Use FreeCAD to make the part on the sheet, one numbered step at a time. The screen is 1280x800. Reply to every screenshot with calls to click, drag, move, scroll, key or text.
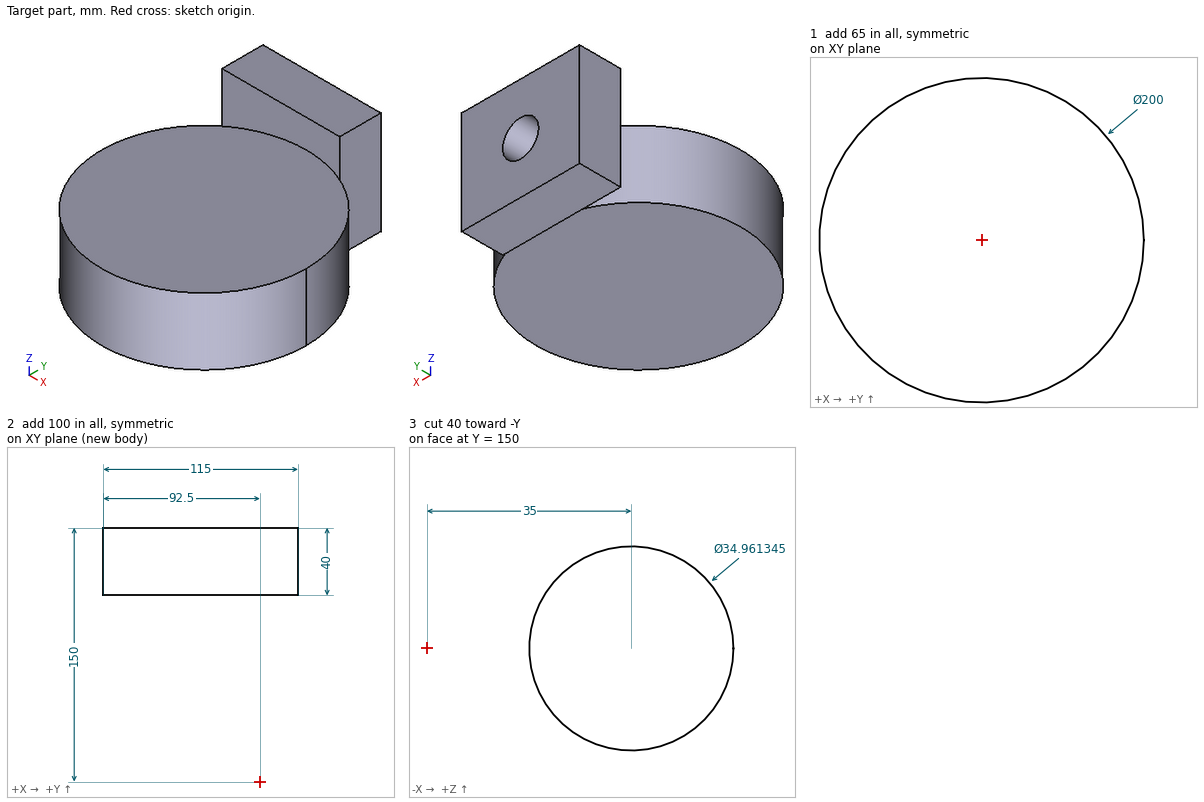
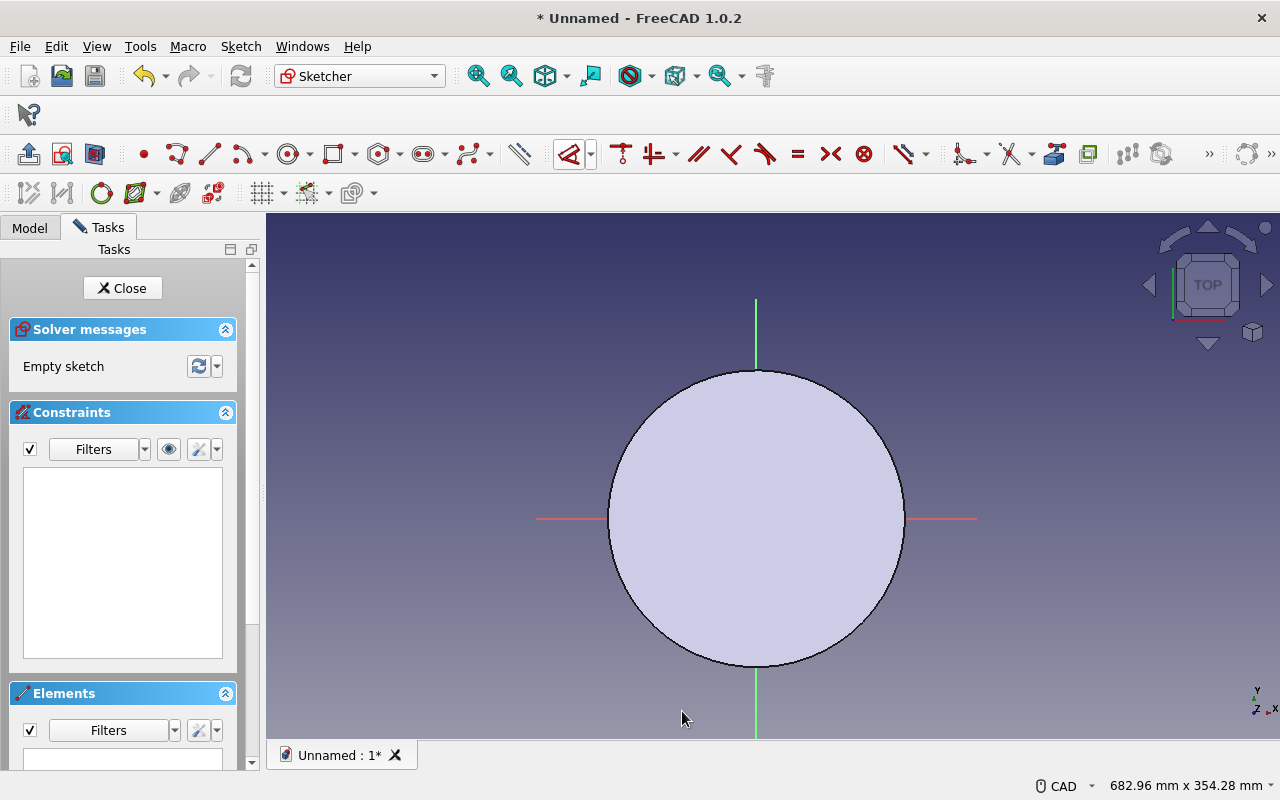
scroll(705, 268, up, 2)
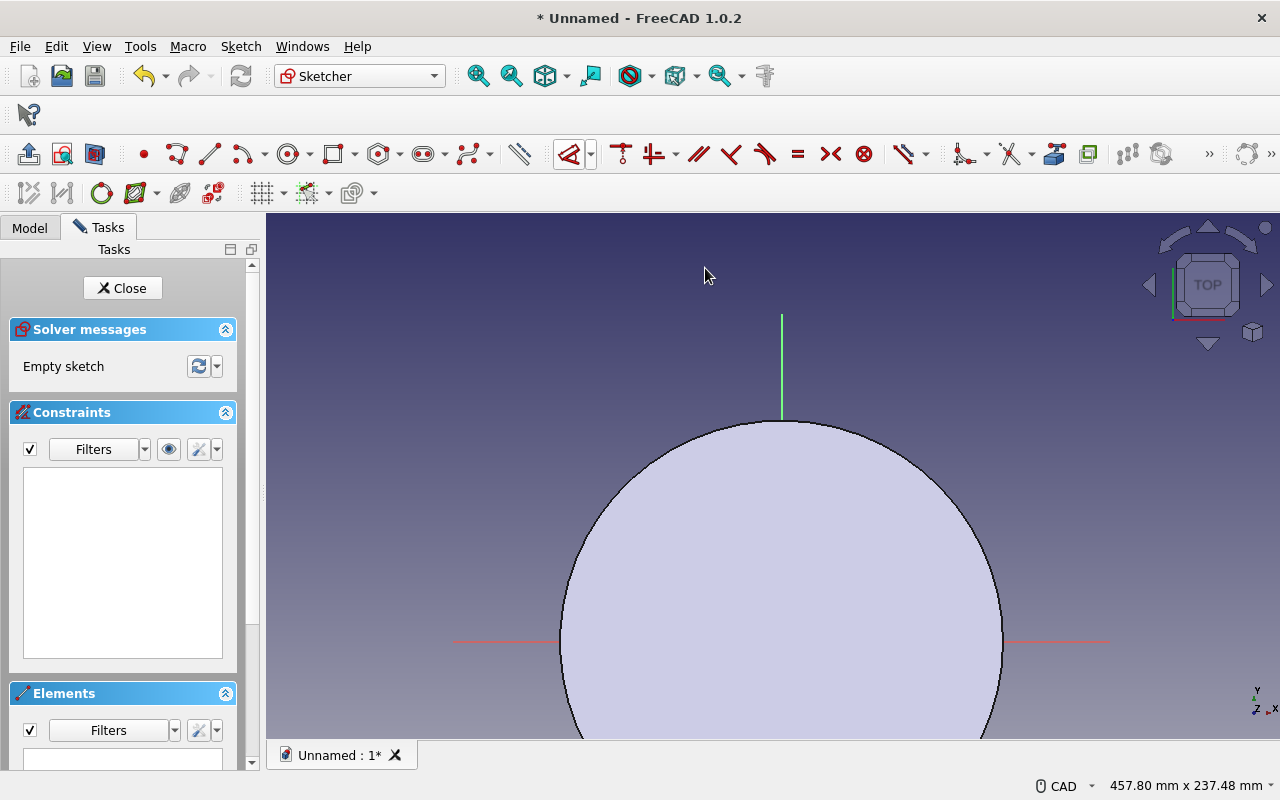
key(g)
key(r)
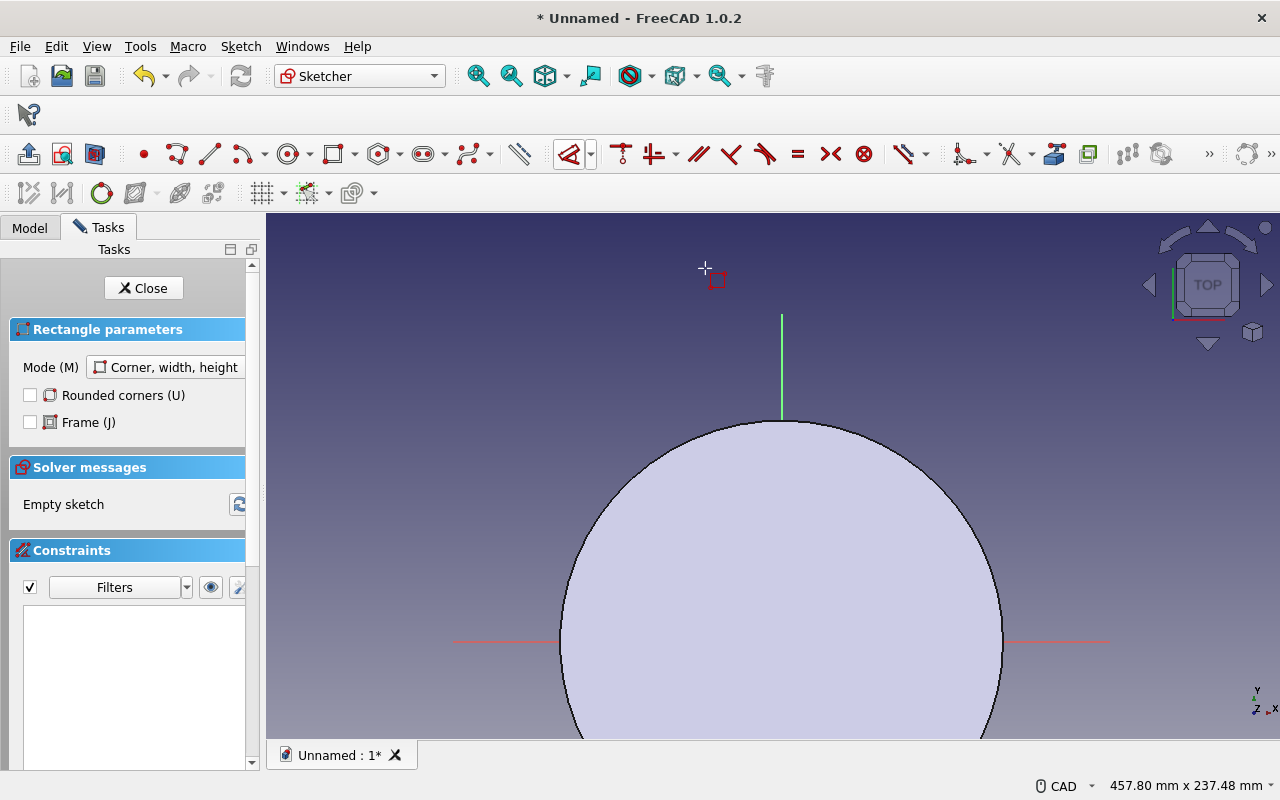
click(577, 310)
move(831, 398)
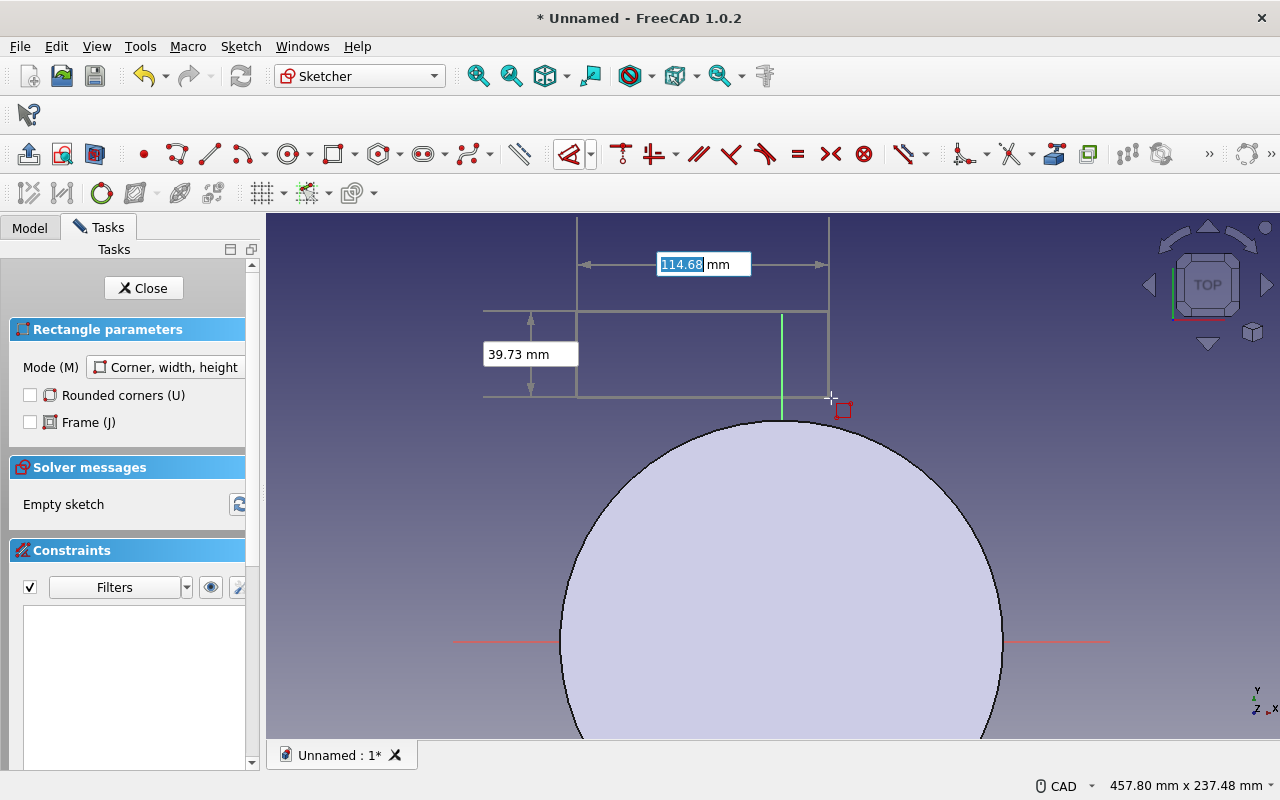
text(115)
key(Tab)
text(40)
key(Return)
key(Escape)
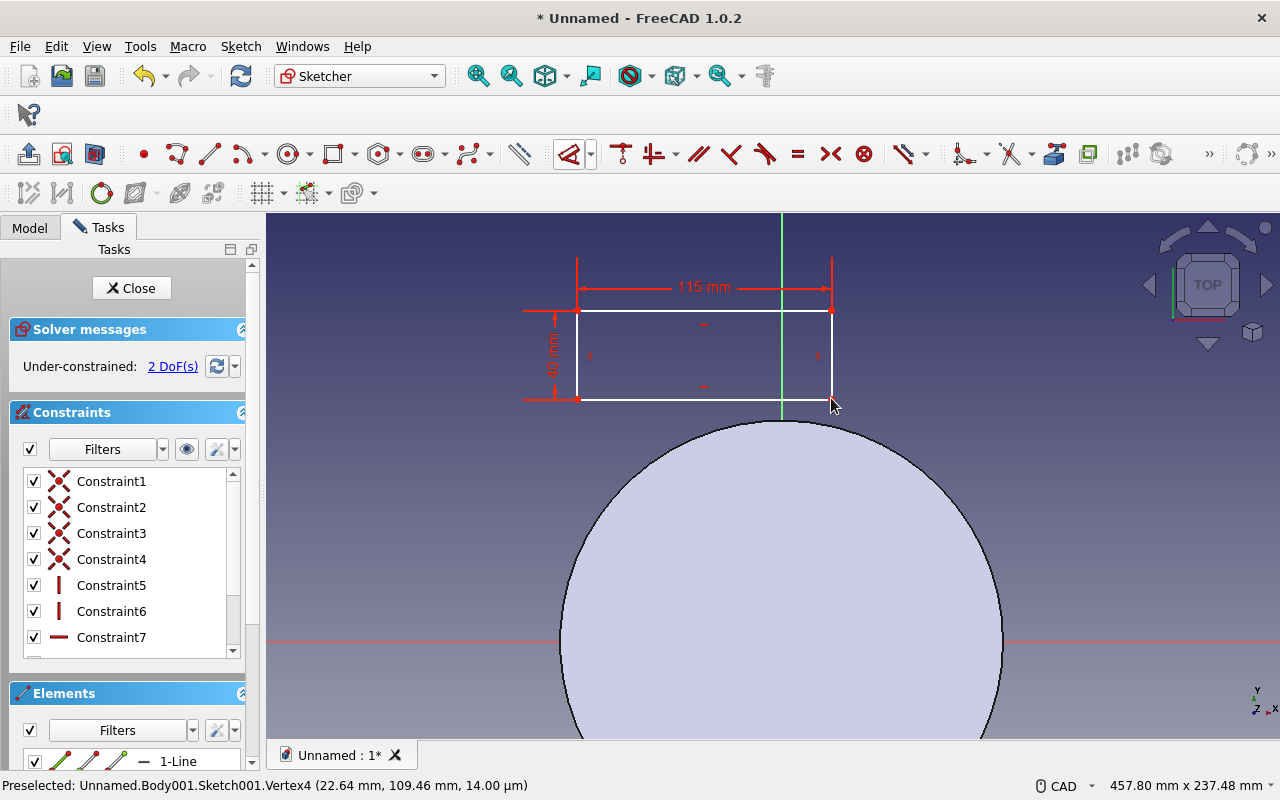
click(568, 154)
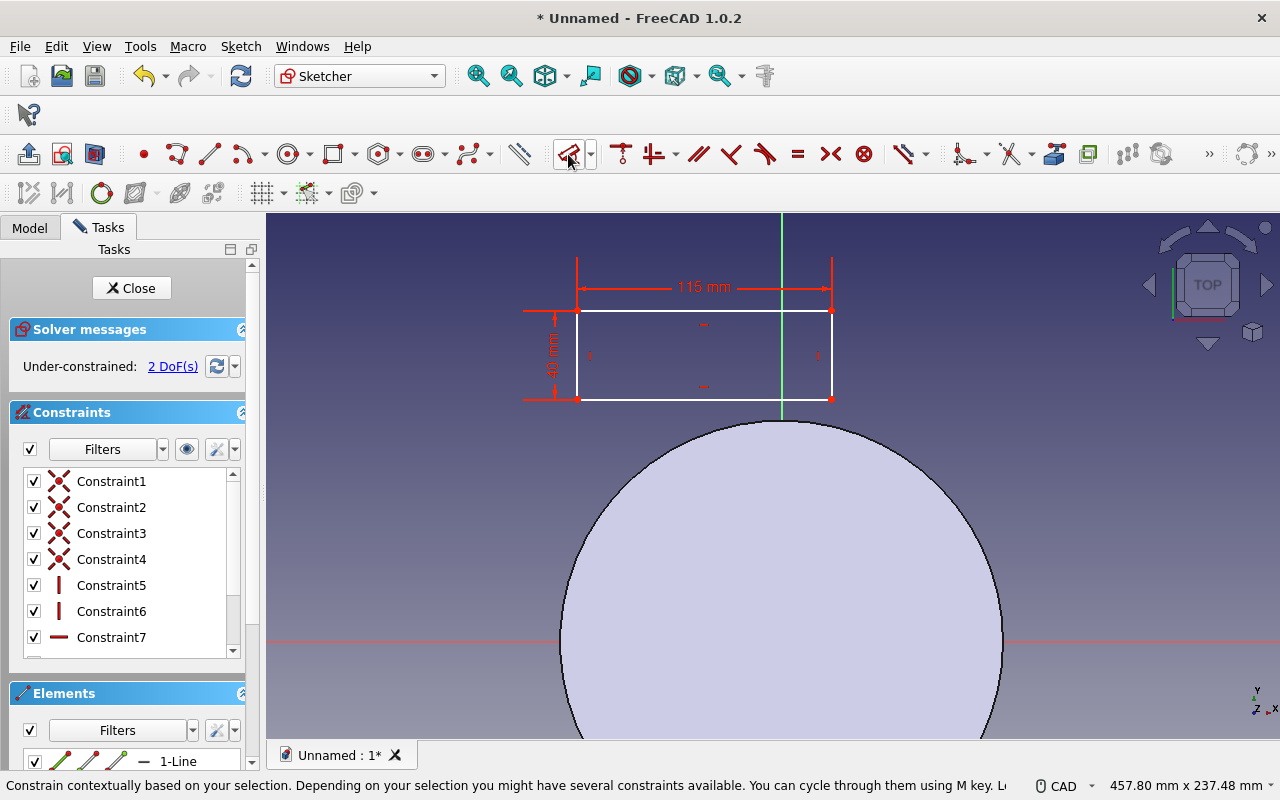
click(577, 311)
click(543, 477)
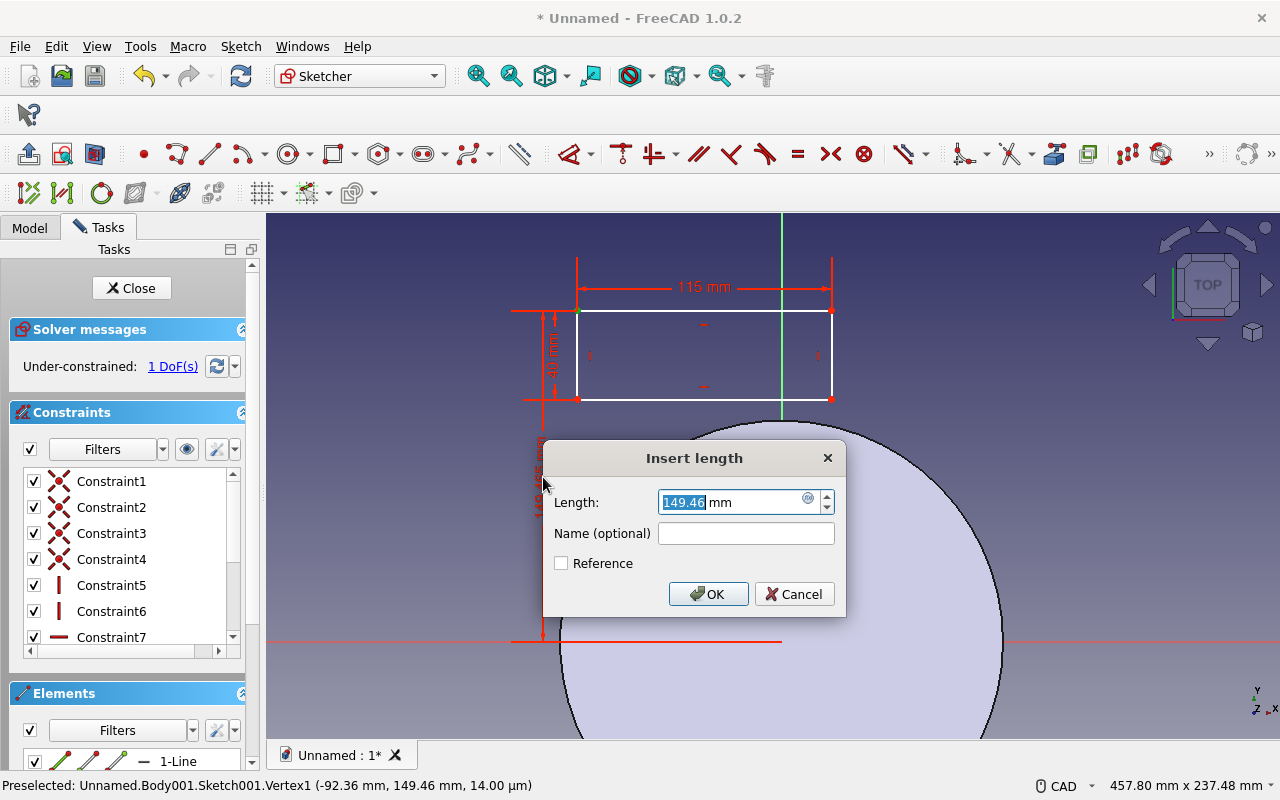
text(150)
key(Return)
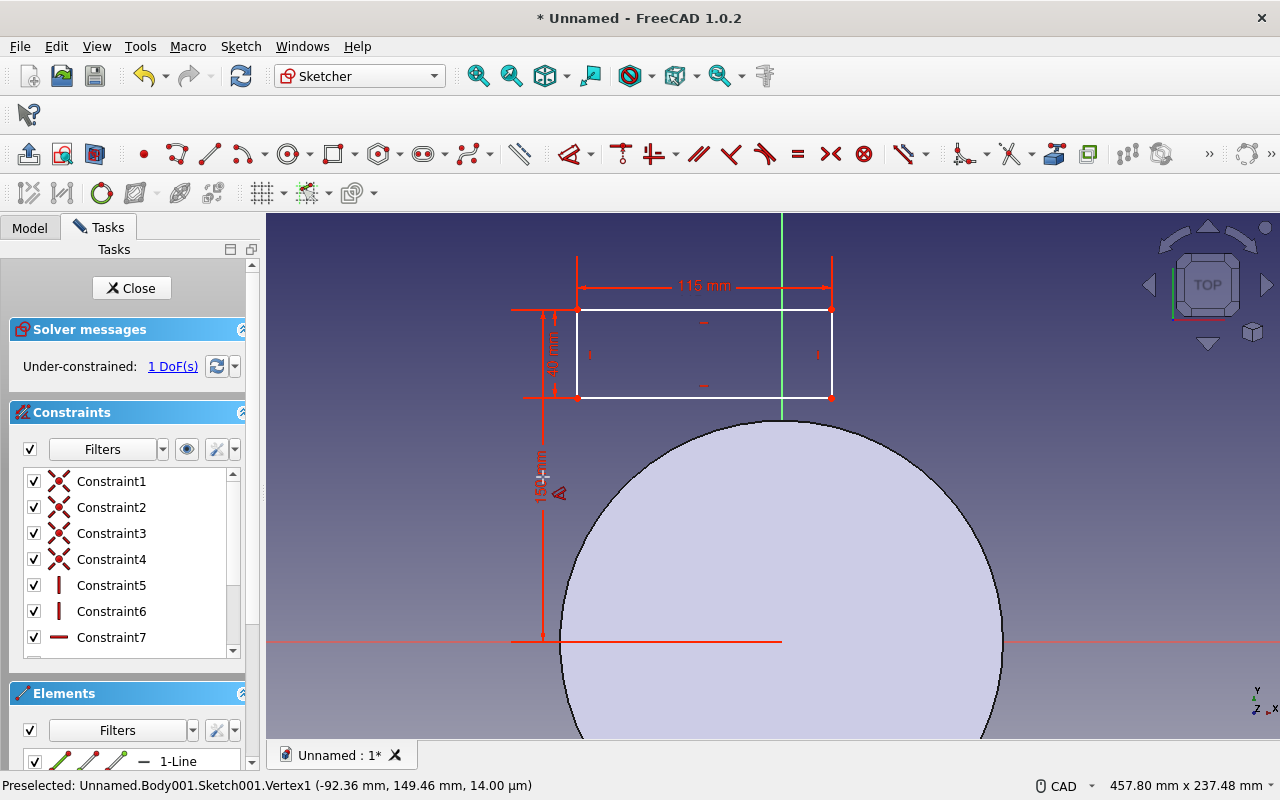
click(577, 310)
click(679, 676)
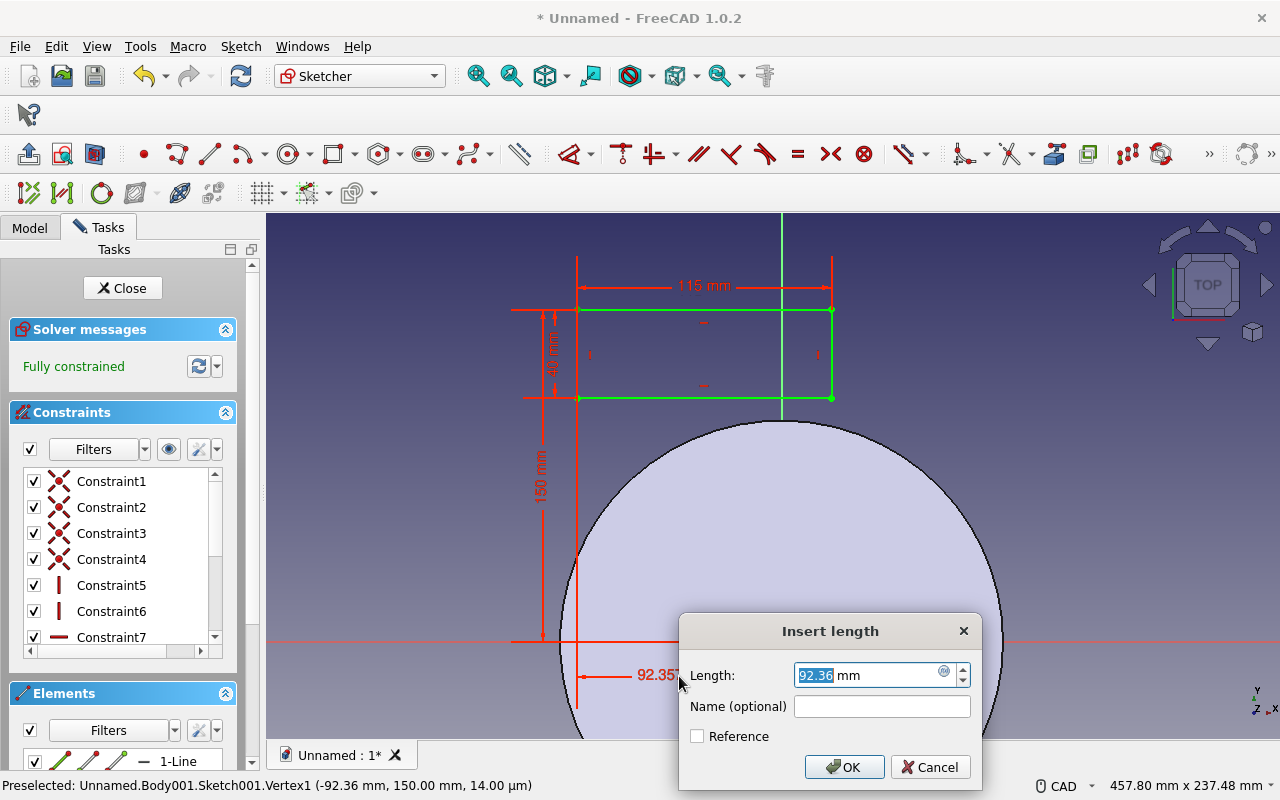
text(92.5)
key(Return)
key(Escape)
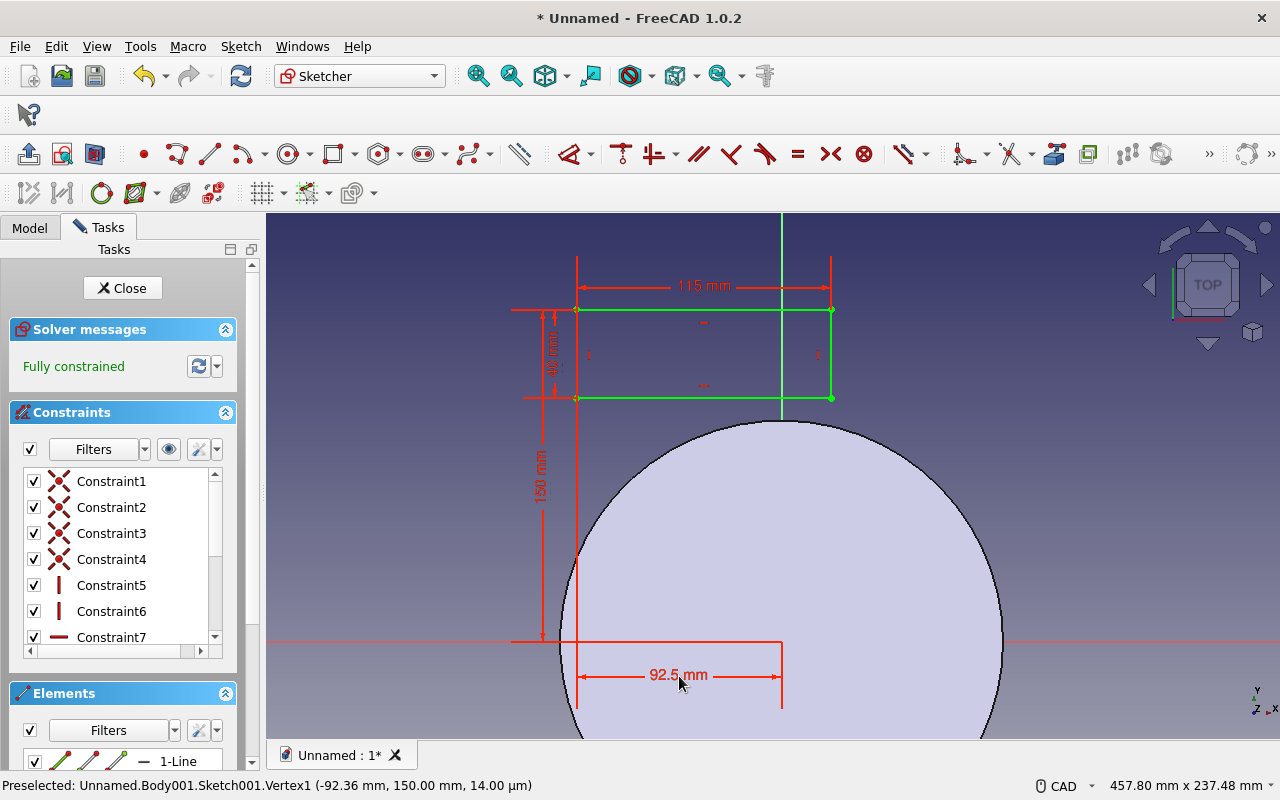
click(123, 288)